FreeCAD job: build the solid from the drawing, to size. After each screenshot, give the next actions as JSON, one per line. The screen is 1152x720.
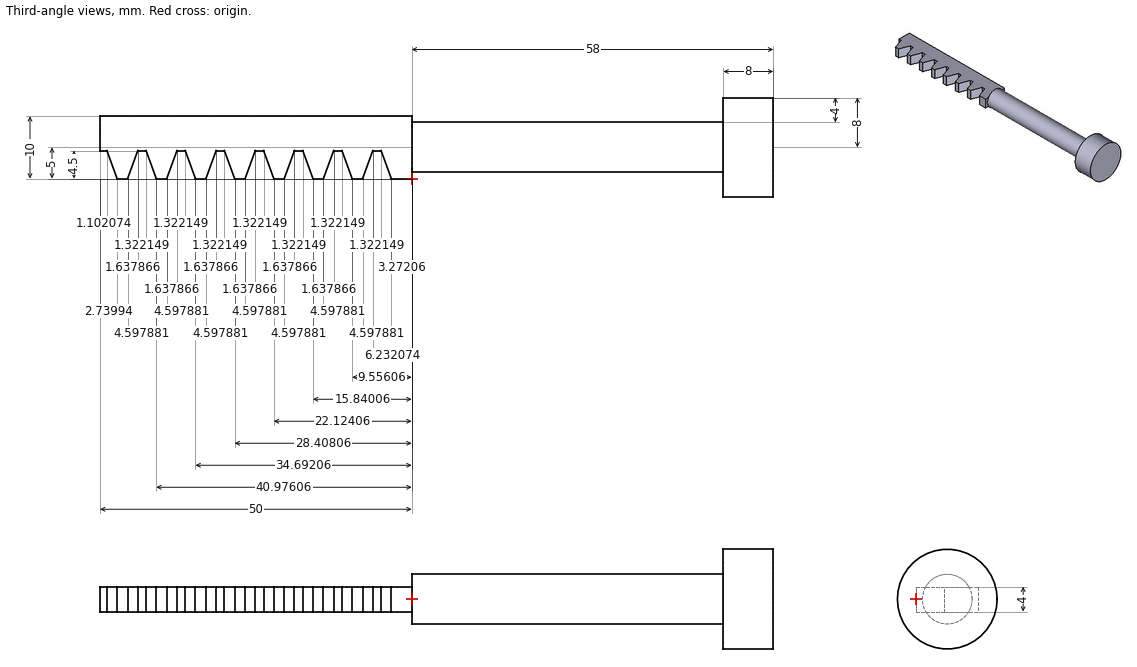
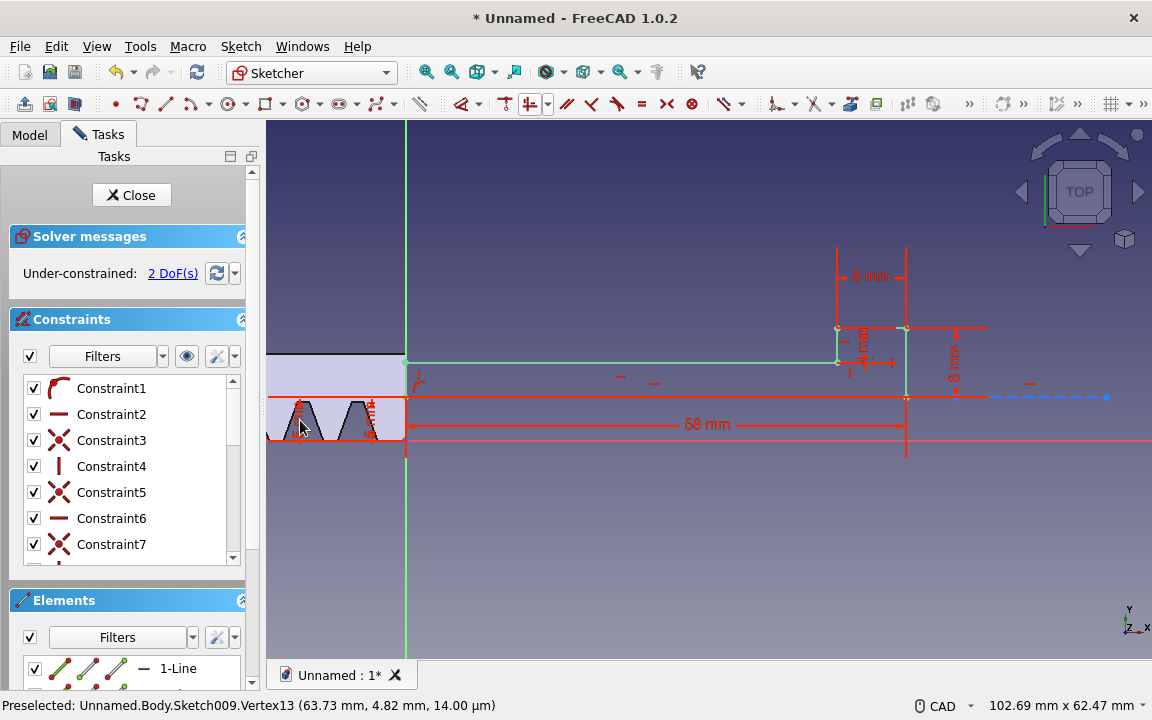
{"action": "left_click", "coordinate": [132, 195]}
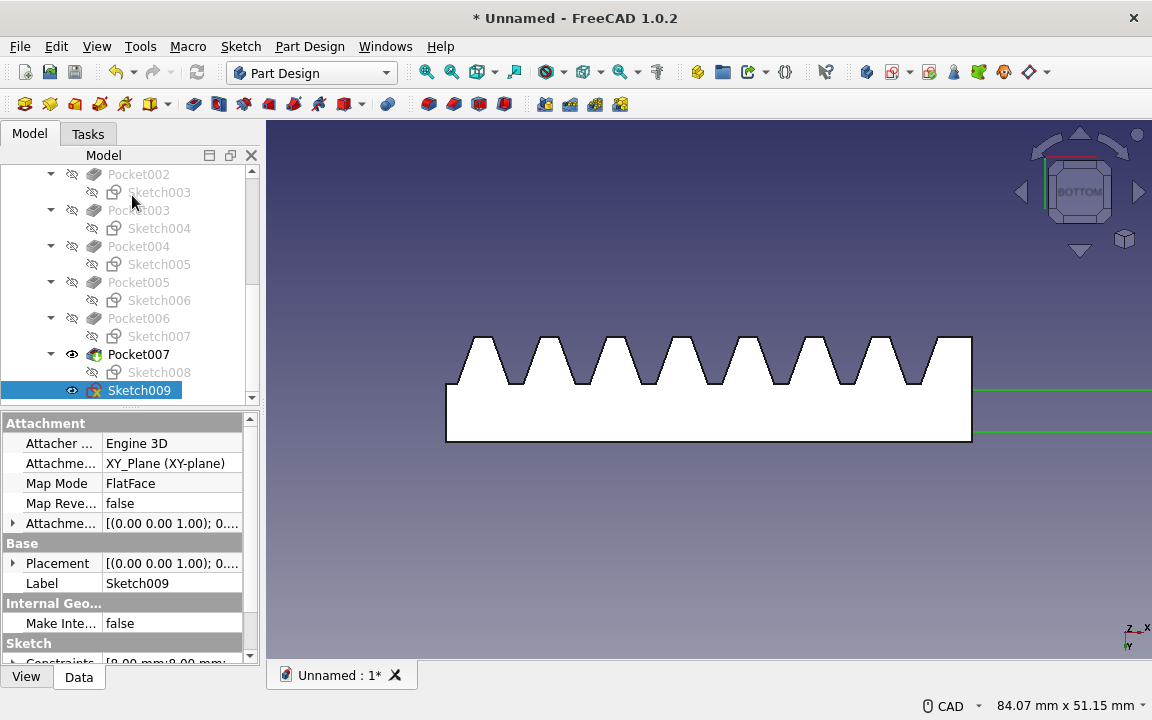
{"action": "left_click", "coordinate": [50, 104]}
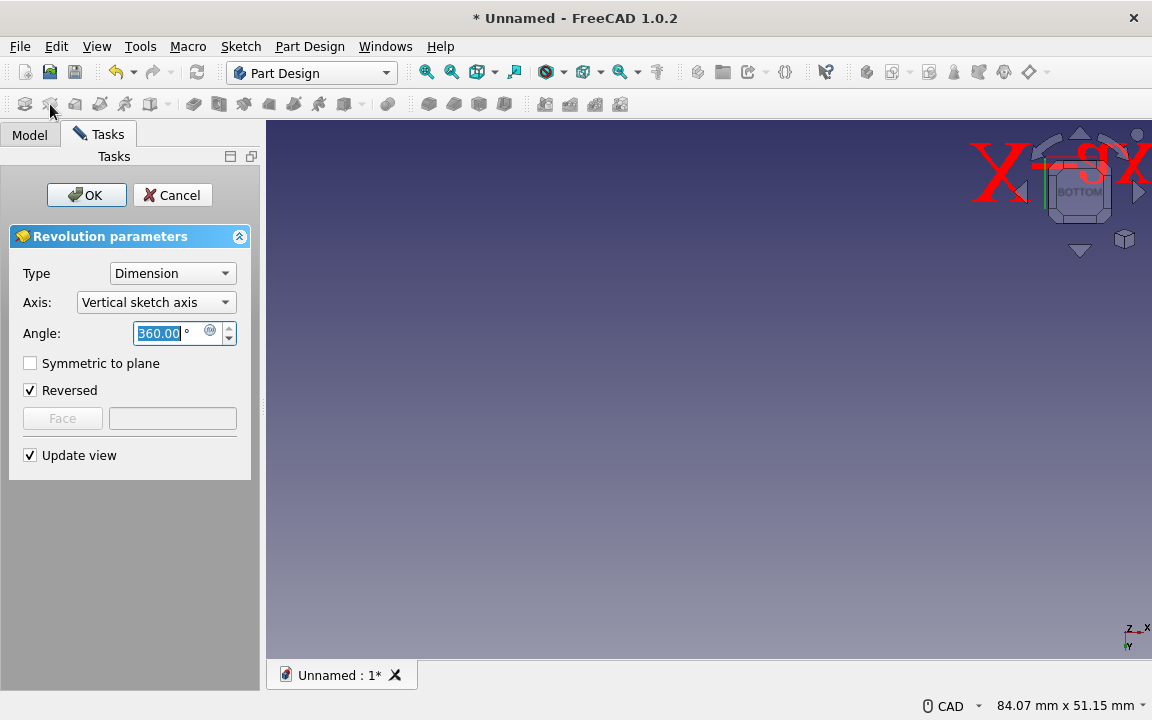
{"action": "left_click", "coordinate": [157, 302]}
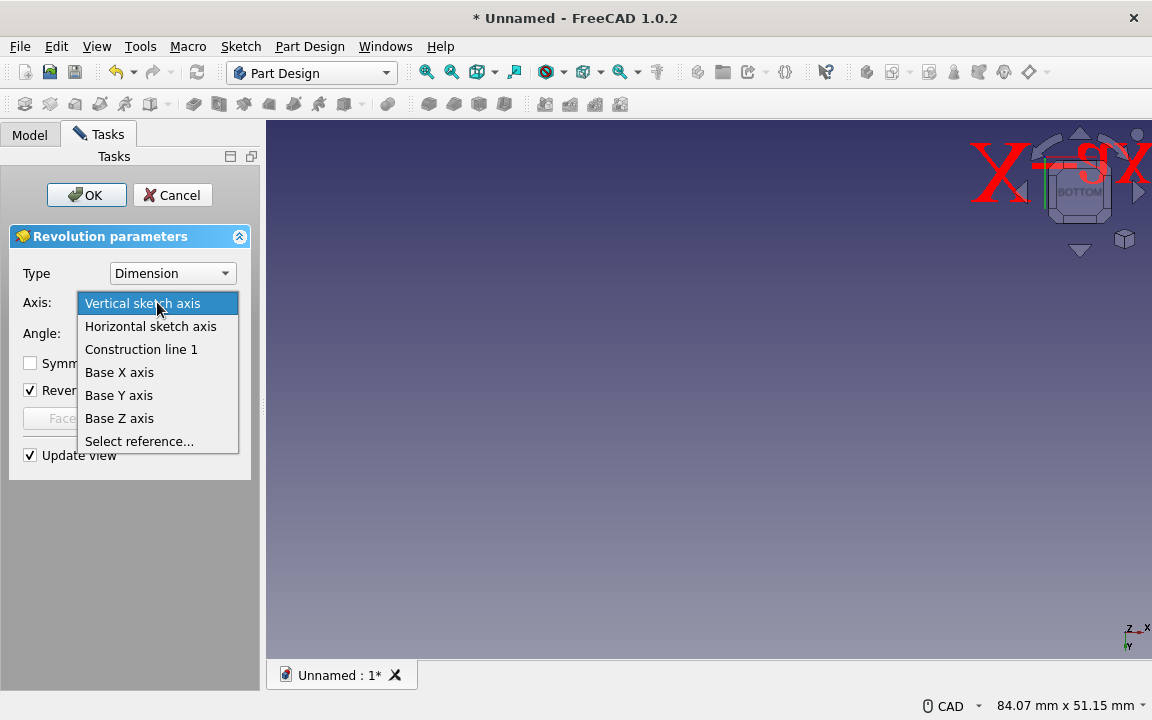
{"action": "left_click", "coordinate": [156, 350]}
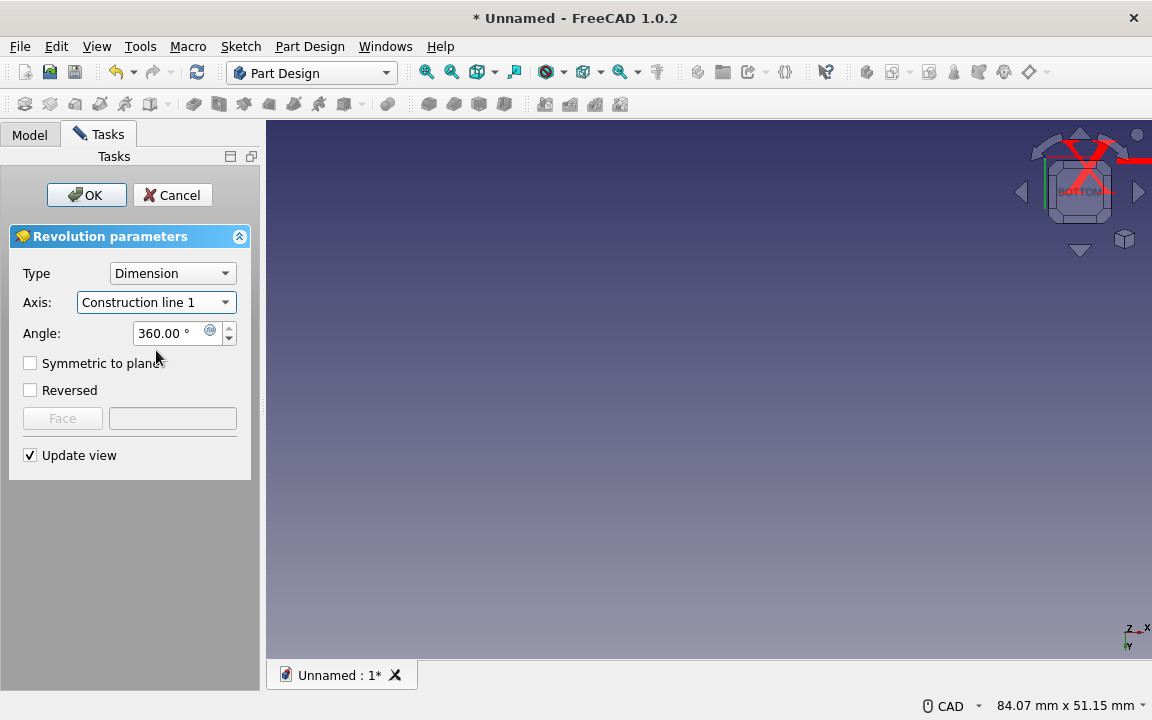
{"action": "left_click", "coordinate": [87, 195]}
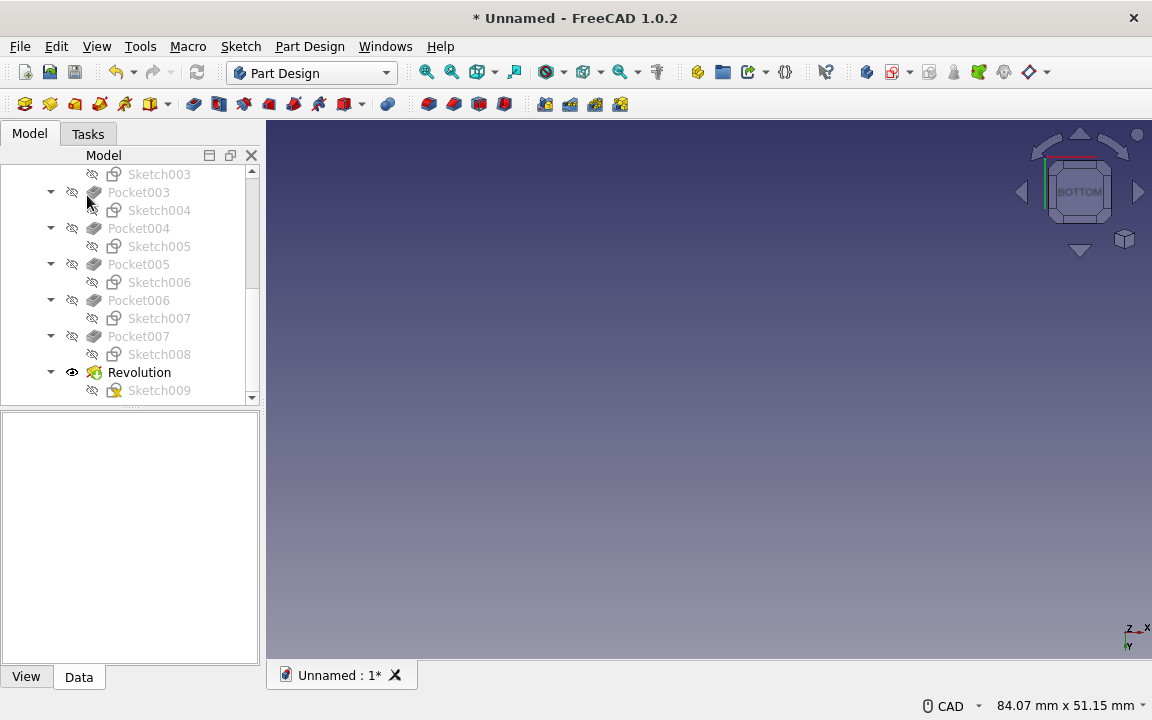
{"action": "key", "text": "0"}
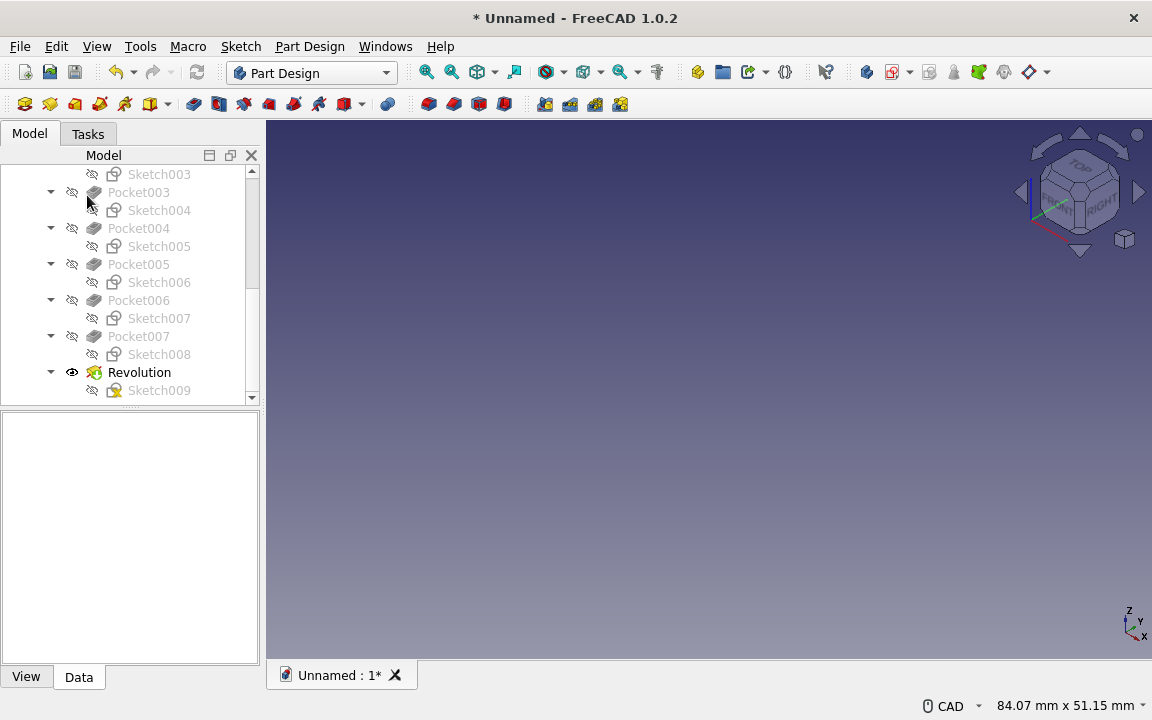
{"action": "left_click", "coordinate": [427, 72]}